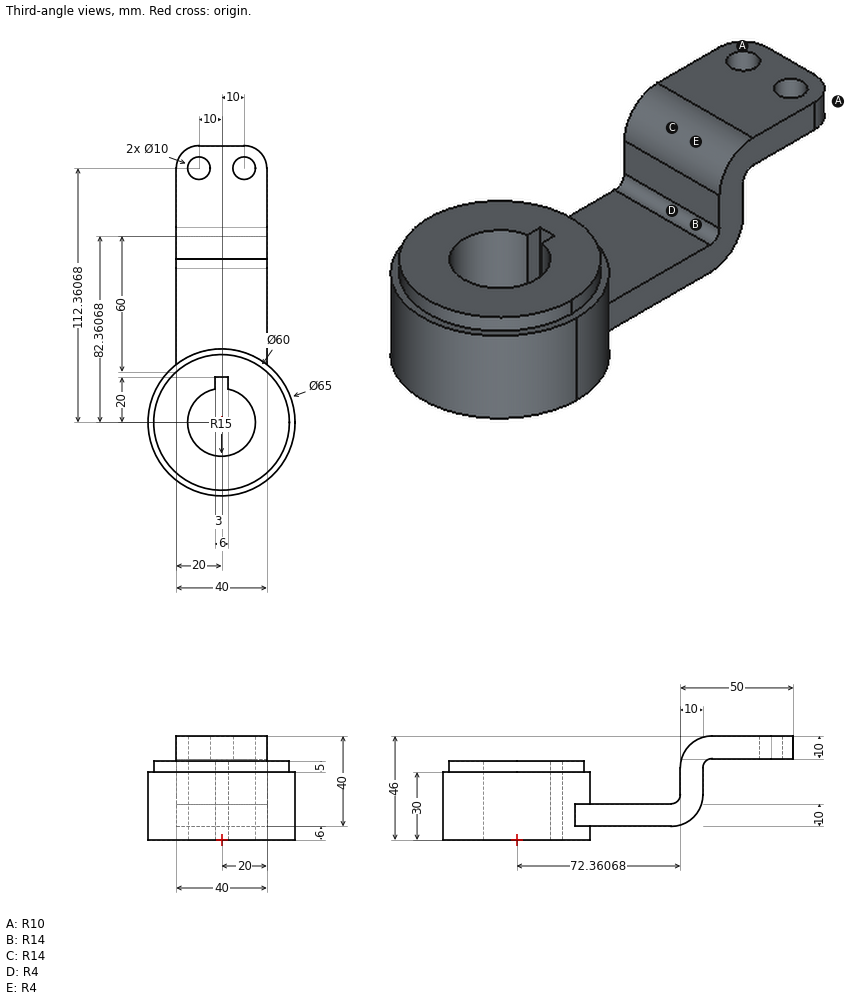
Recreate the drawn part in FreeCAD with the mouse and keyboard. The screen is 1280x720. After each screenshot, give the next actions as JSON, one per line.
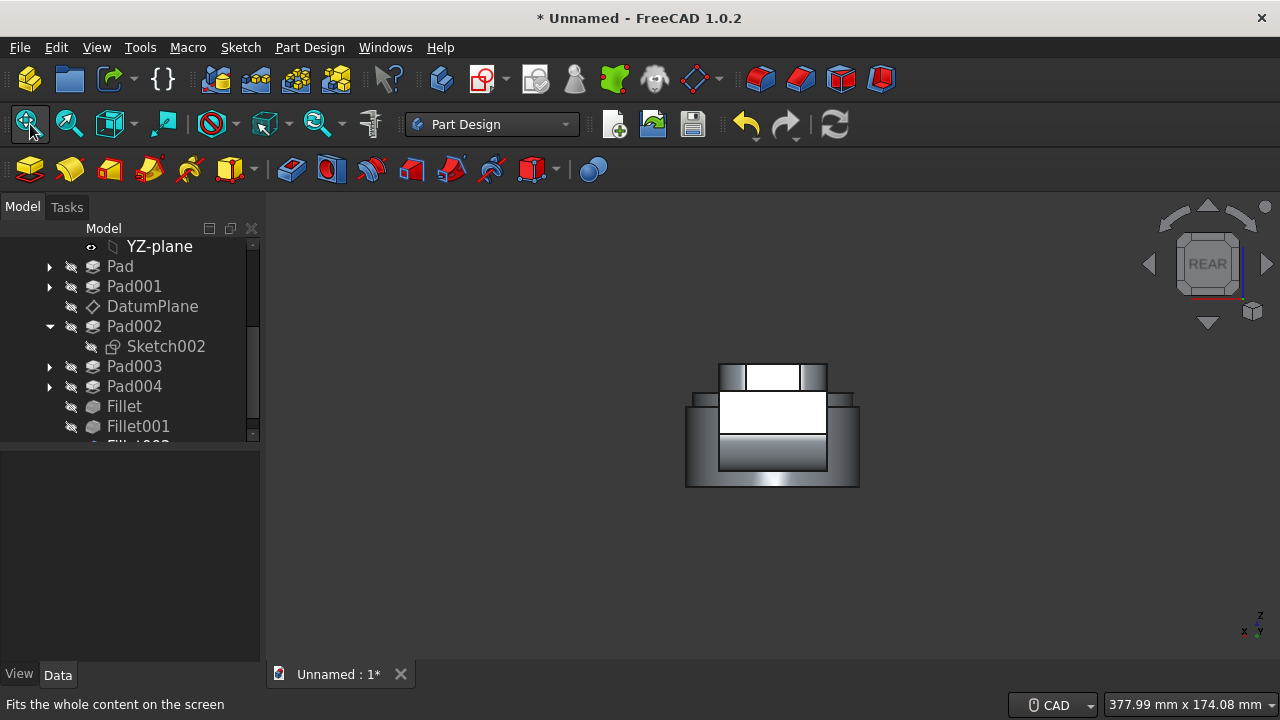
{"action": "key", "text": "6"}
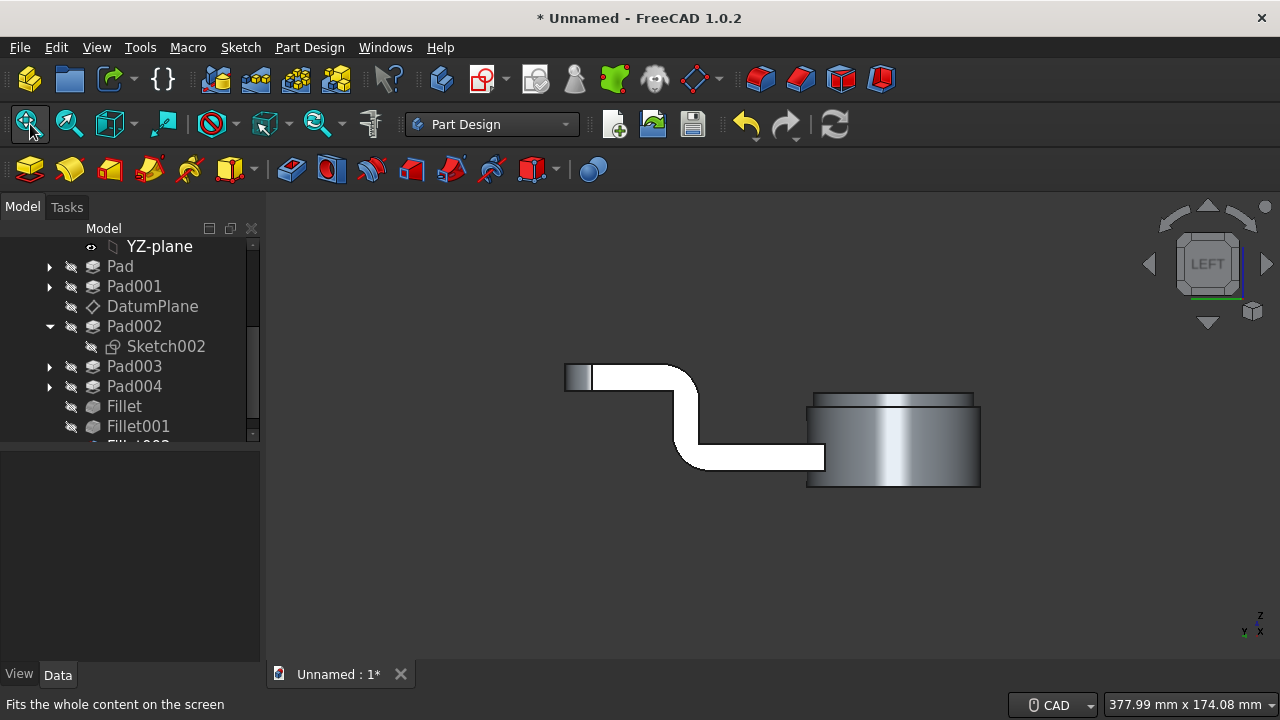
{"action": "key", "text": "v f"}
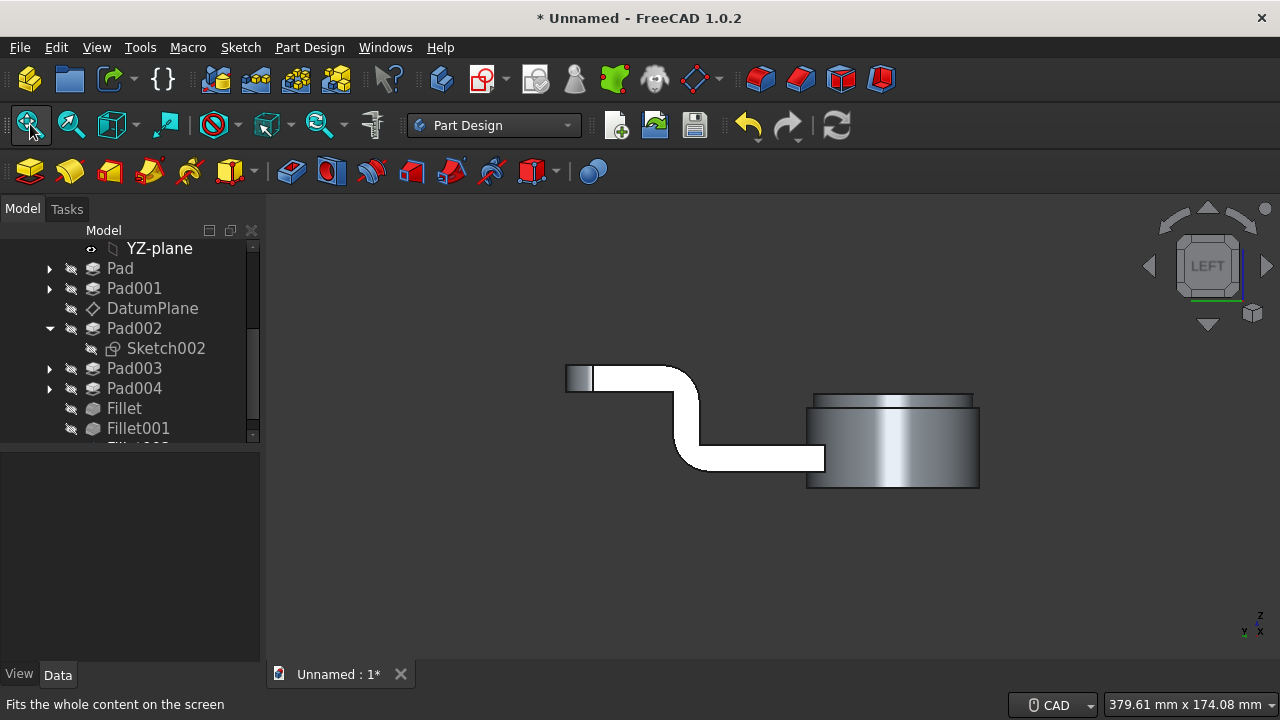
{"action": "key", "text": "v 3"}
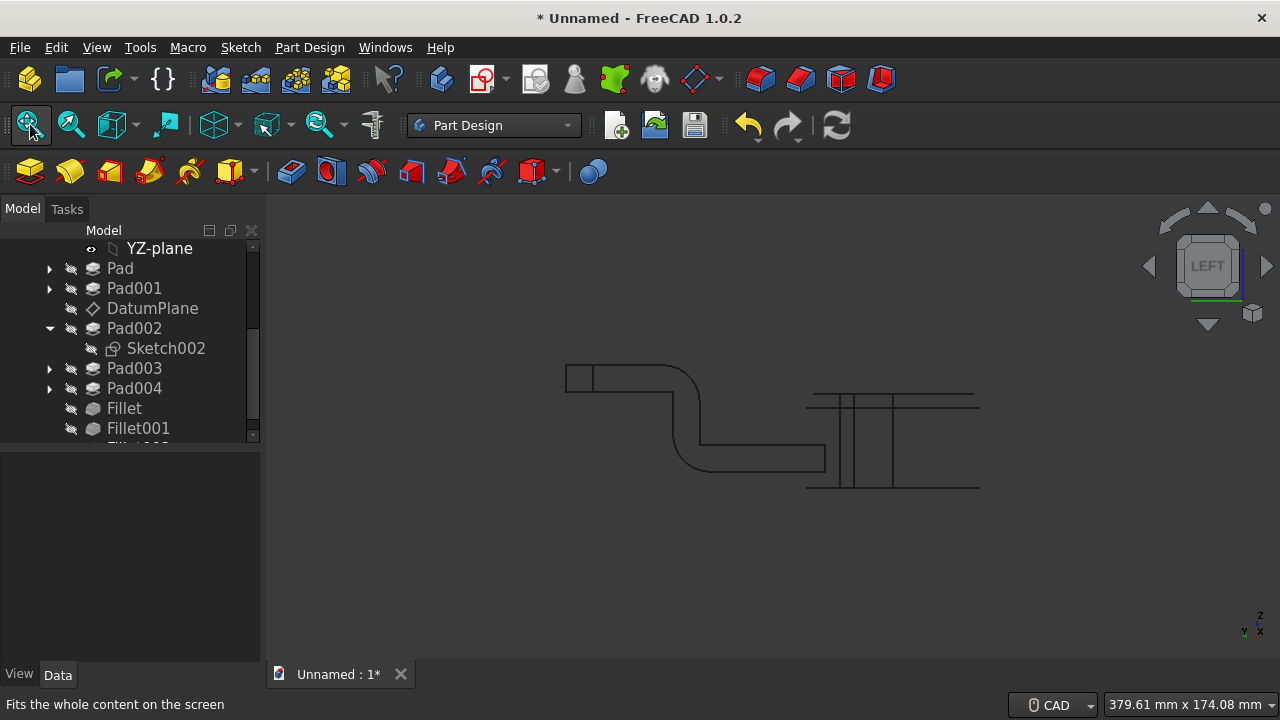
{"action": "key", "text": "0"}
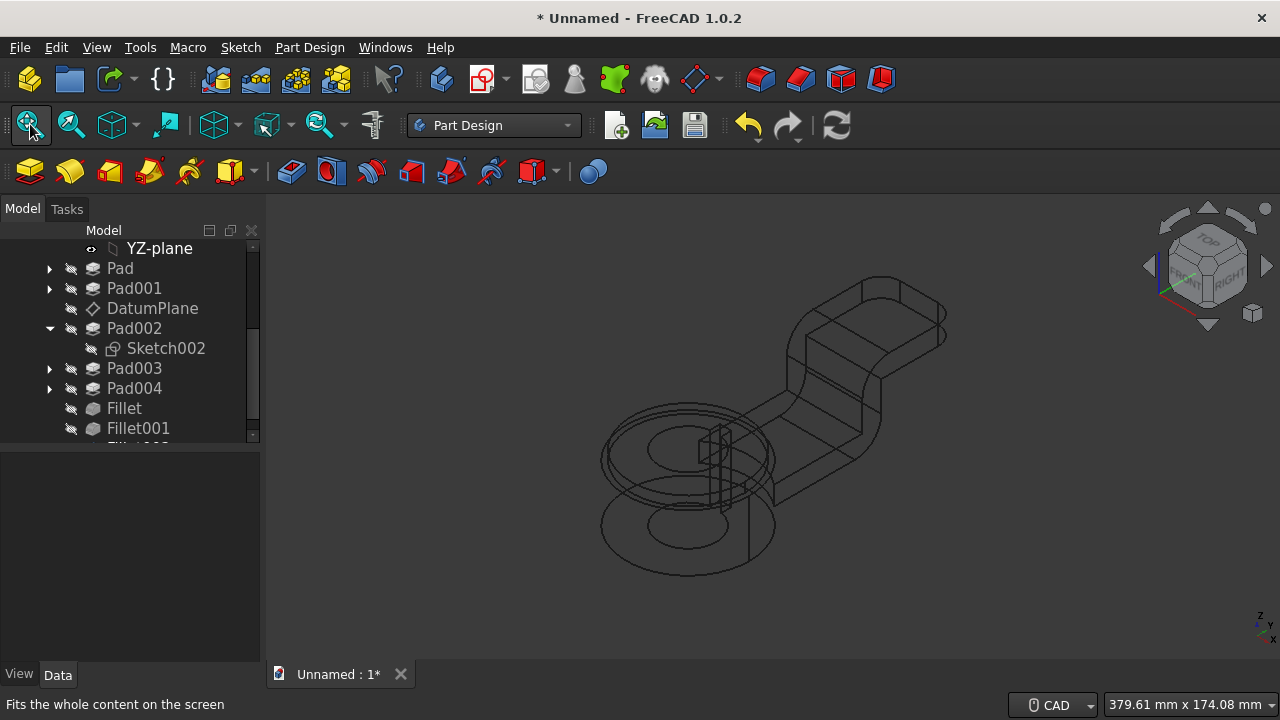
{"action": "left_click", "coordinate": [825, 411]}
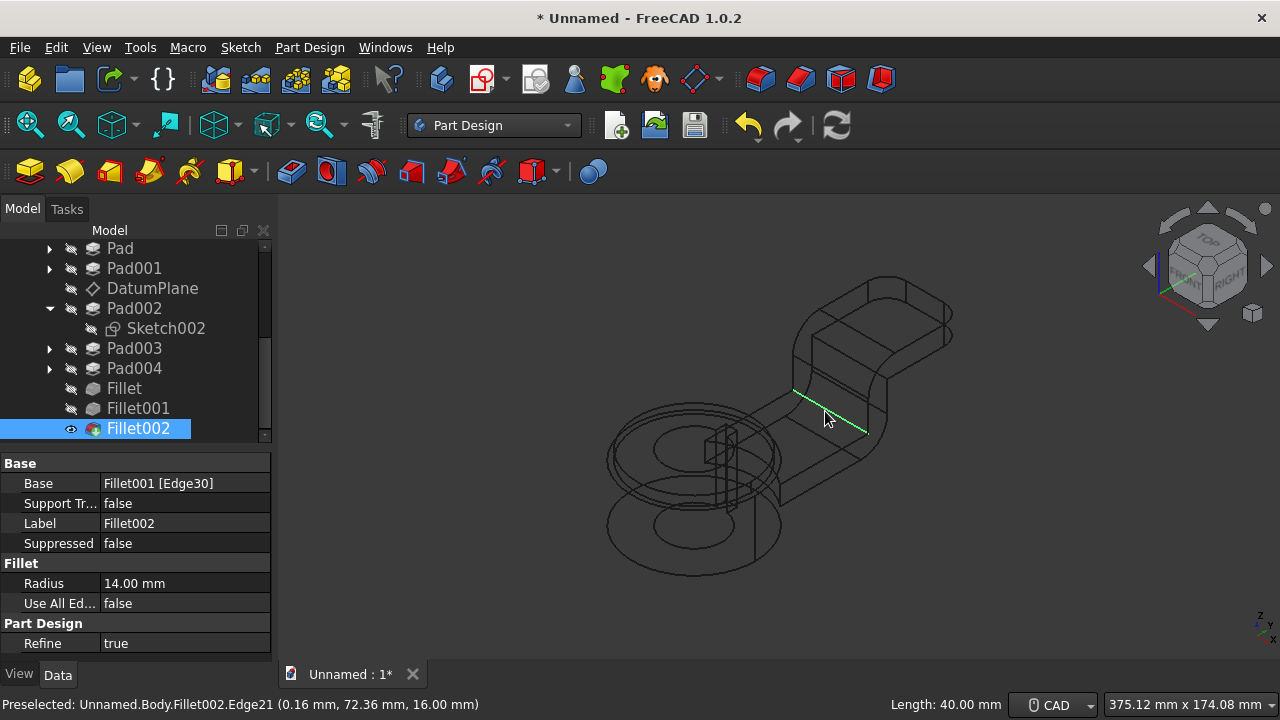
{"action": "key", "text": "v 1"}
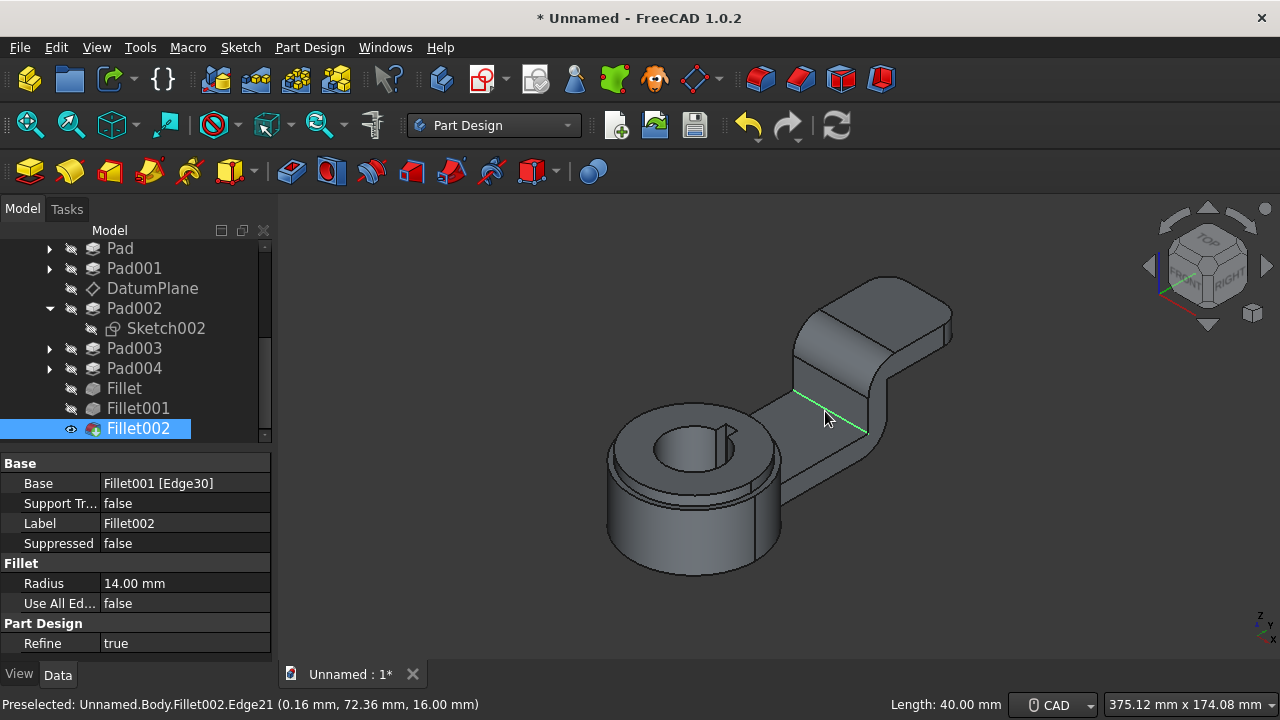
{"action": "left_click", "coordinate": [762, 80]}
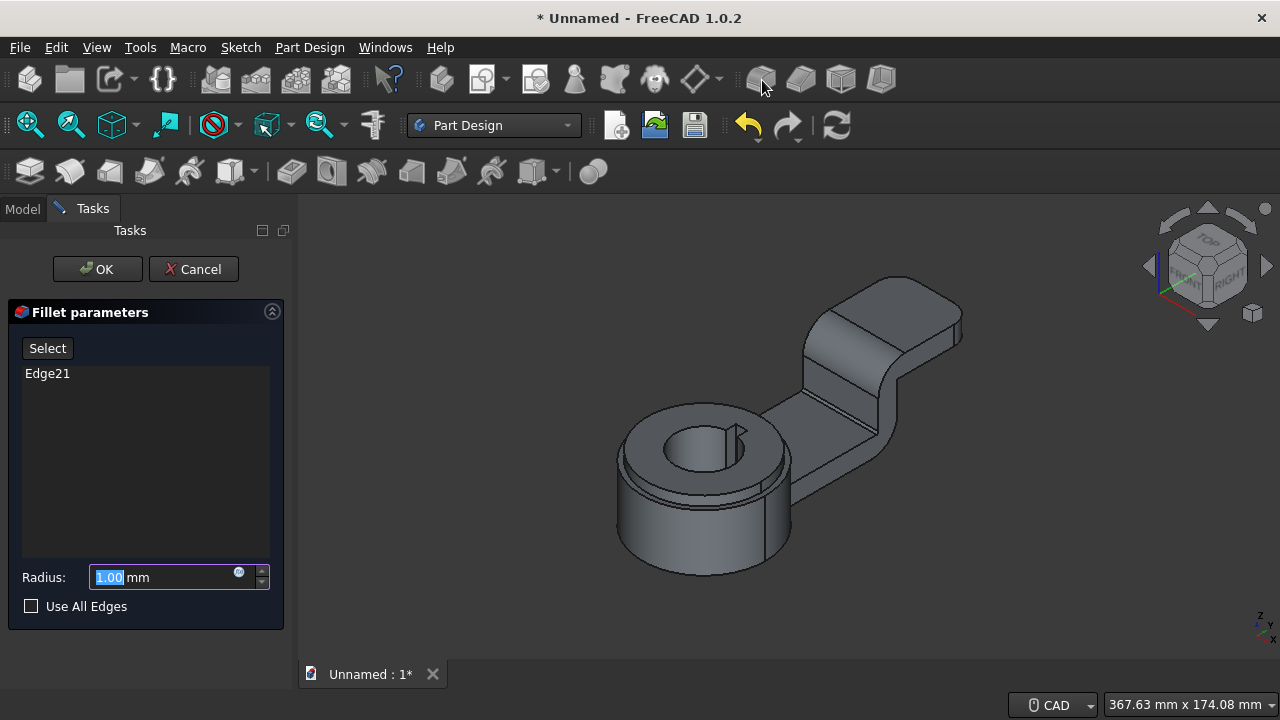
{"action": "type", "text": "4"}
{"action": "key", "text": "Tab"}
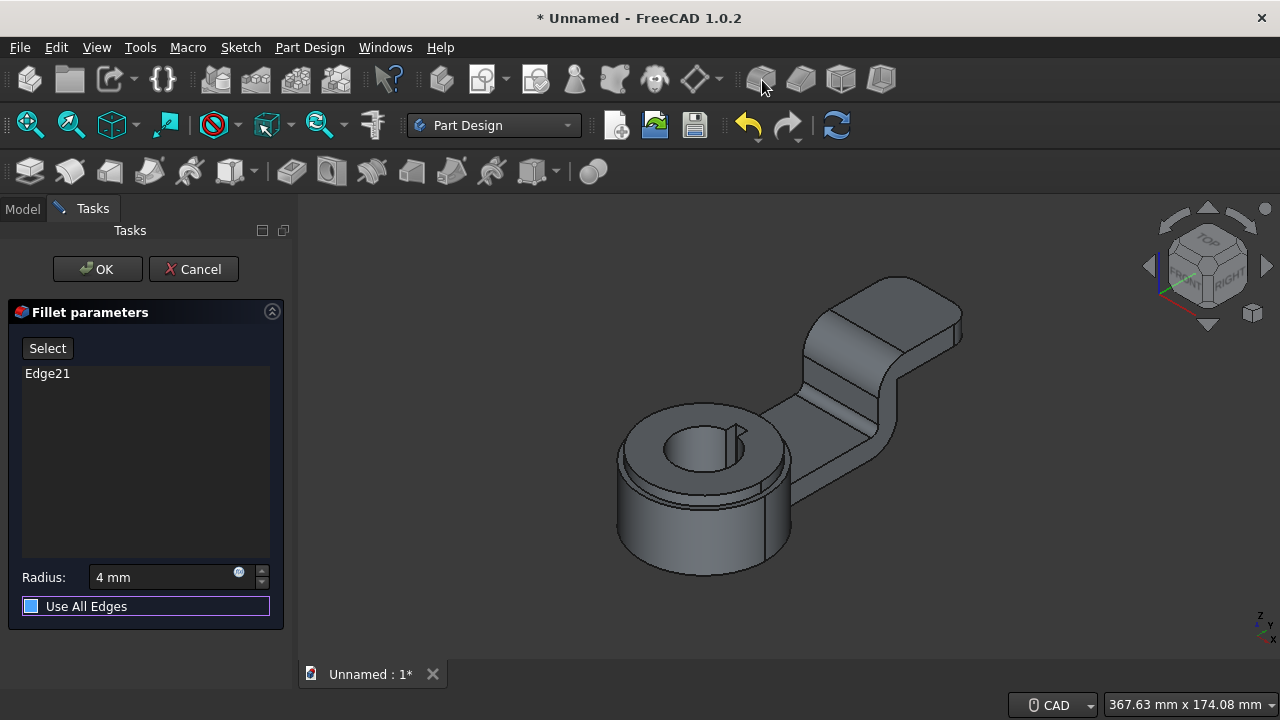
{"action": "left_click", "coordinate": [98, 269]}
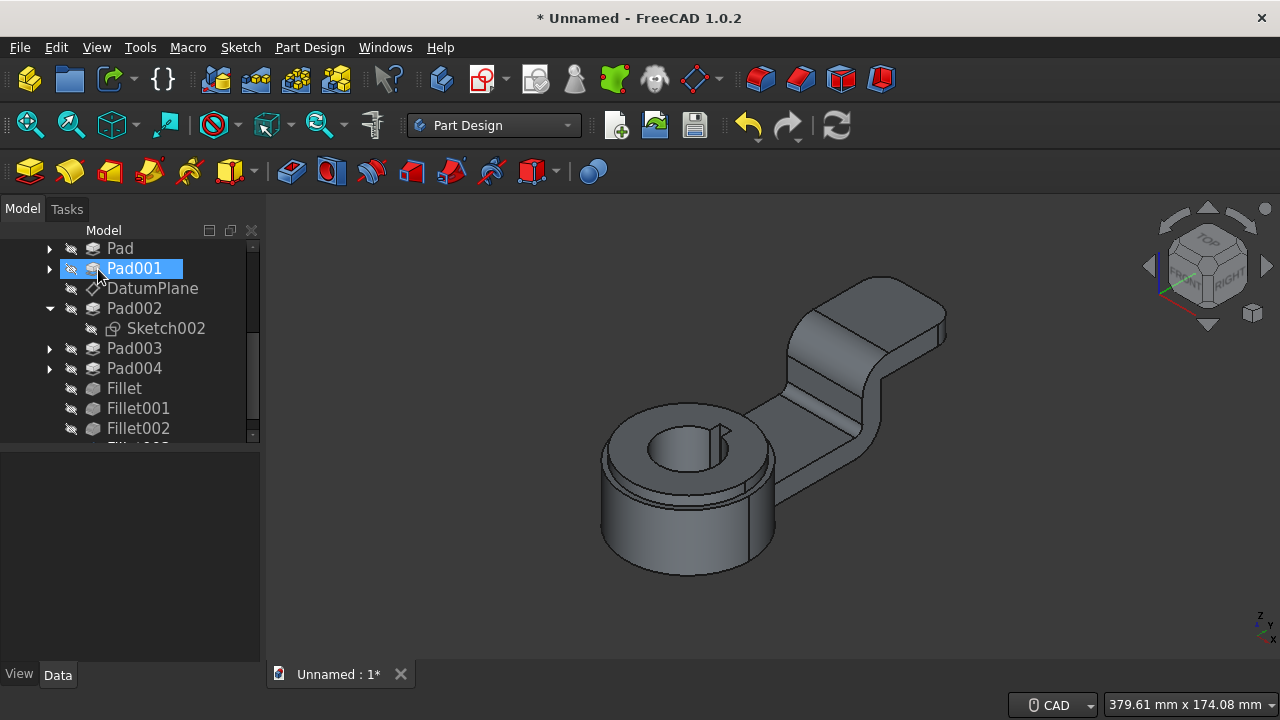
{"action": "key", "text": "2"}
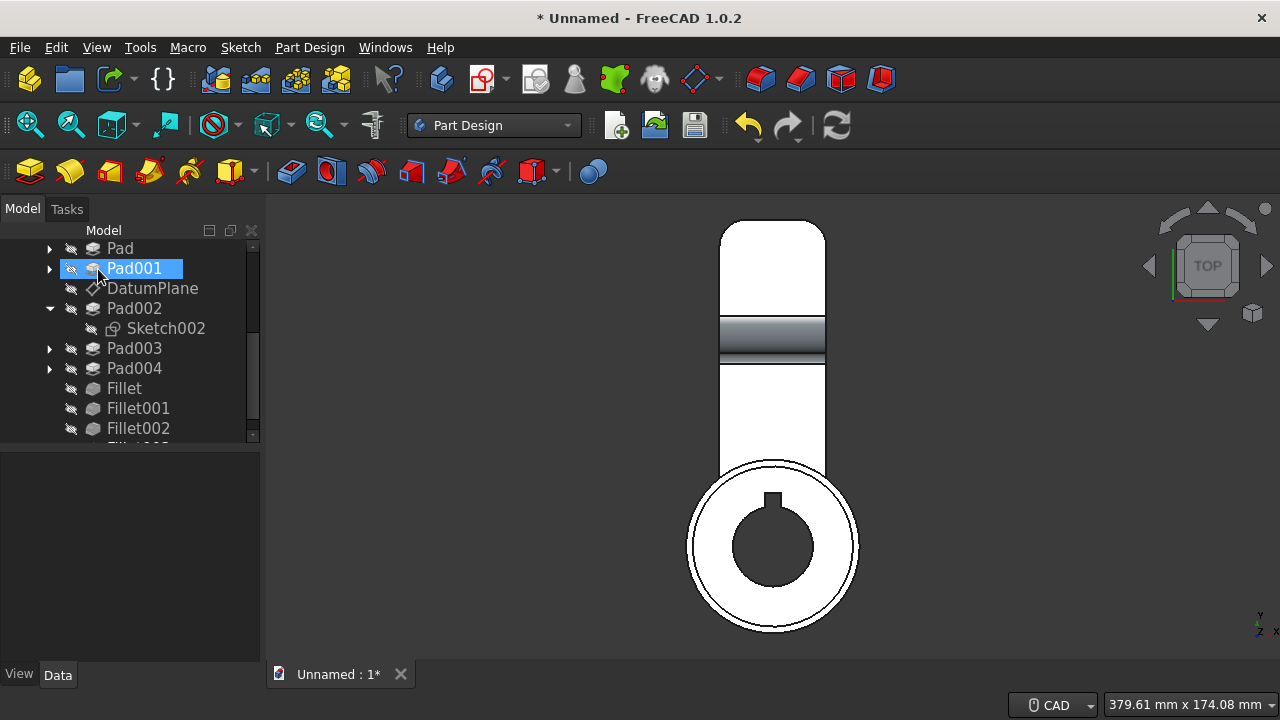
{"action": "key", "text": "0"}